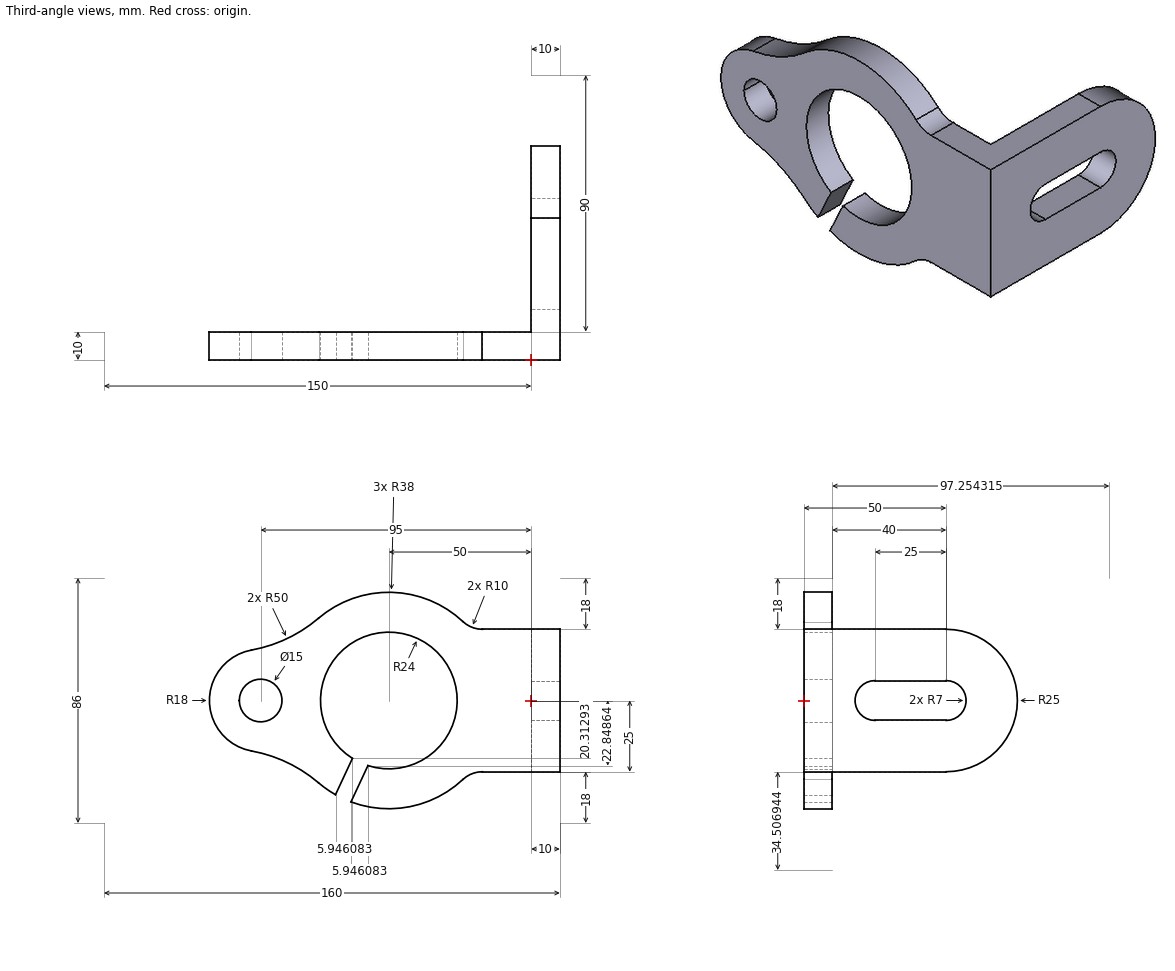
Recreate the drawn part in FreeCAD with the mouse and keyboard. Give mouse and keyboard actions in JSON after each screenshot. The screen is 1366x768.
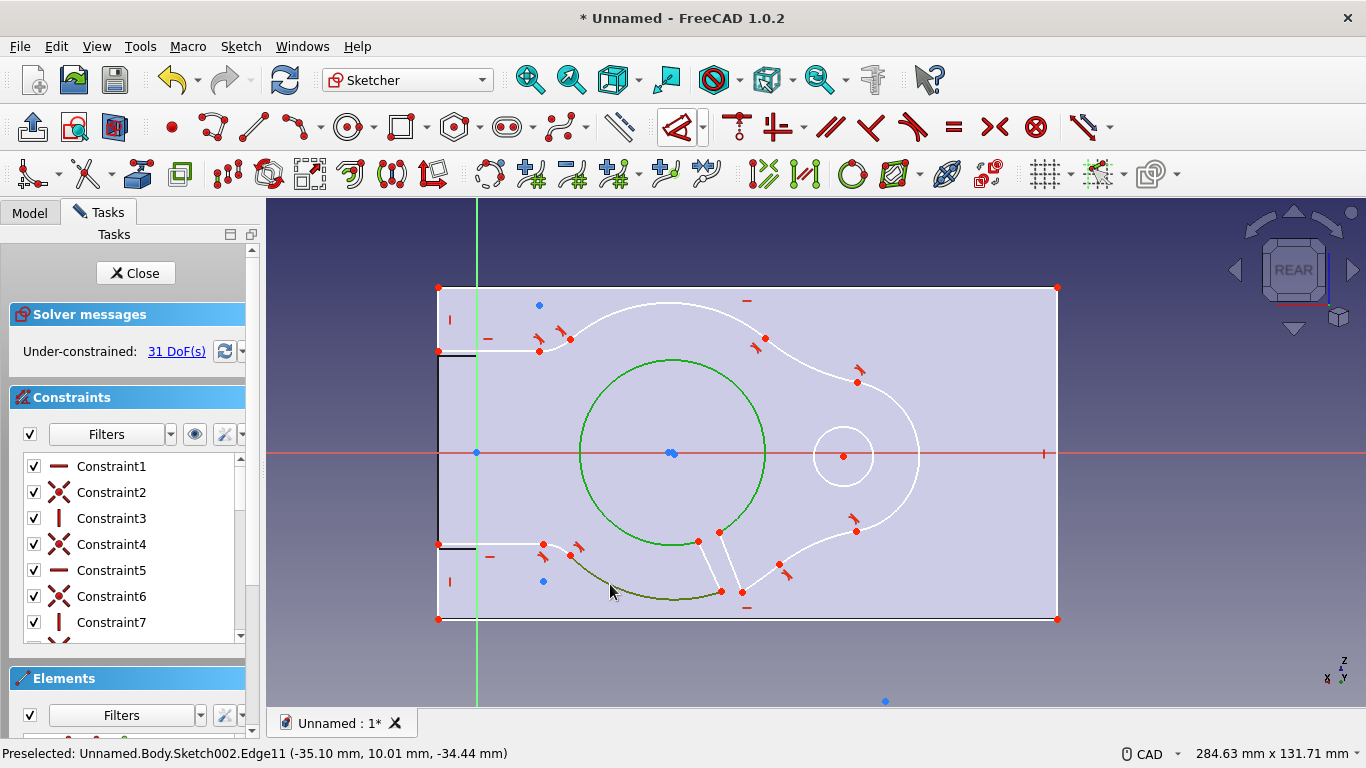
{"action": "left_click", "coordinate": [737, 128]}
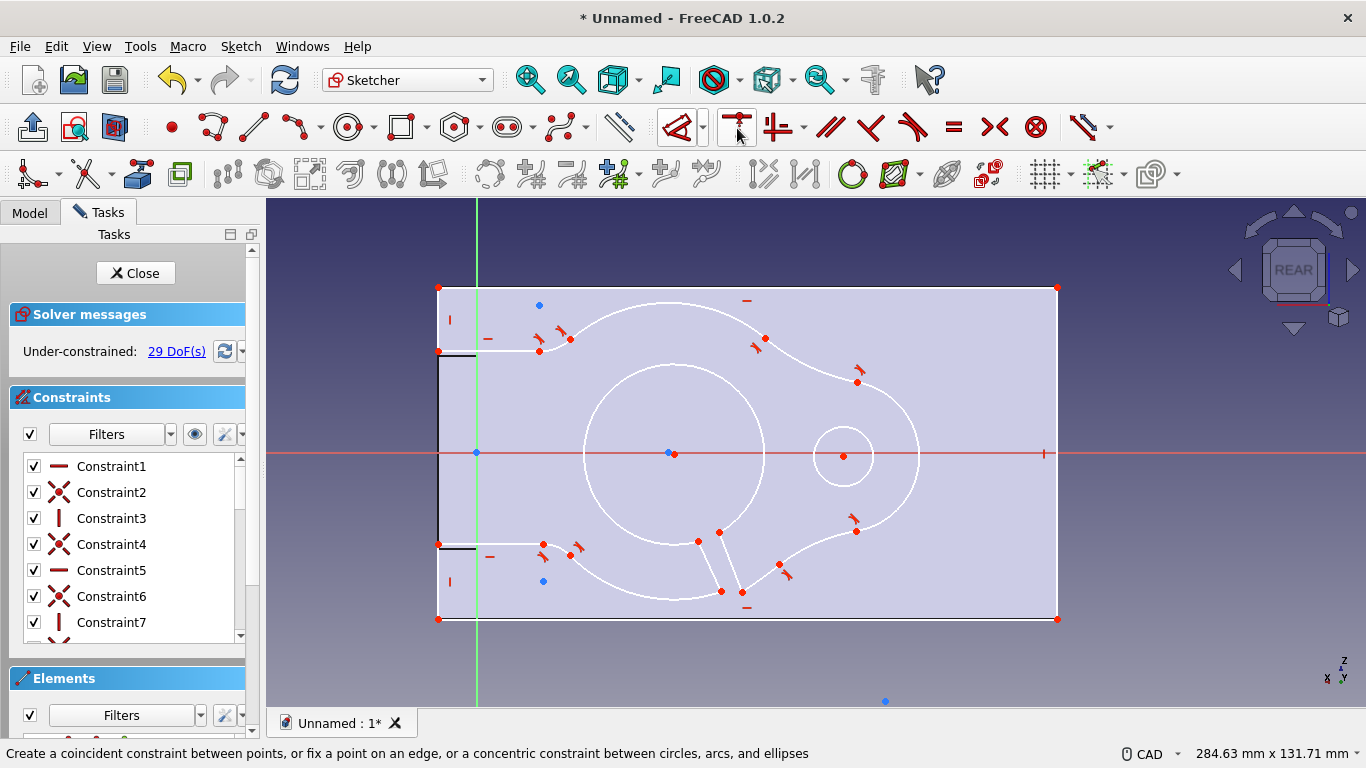
{"action": "left_click", "coordinate": [740, 392]}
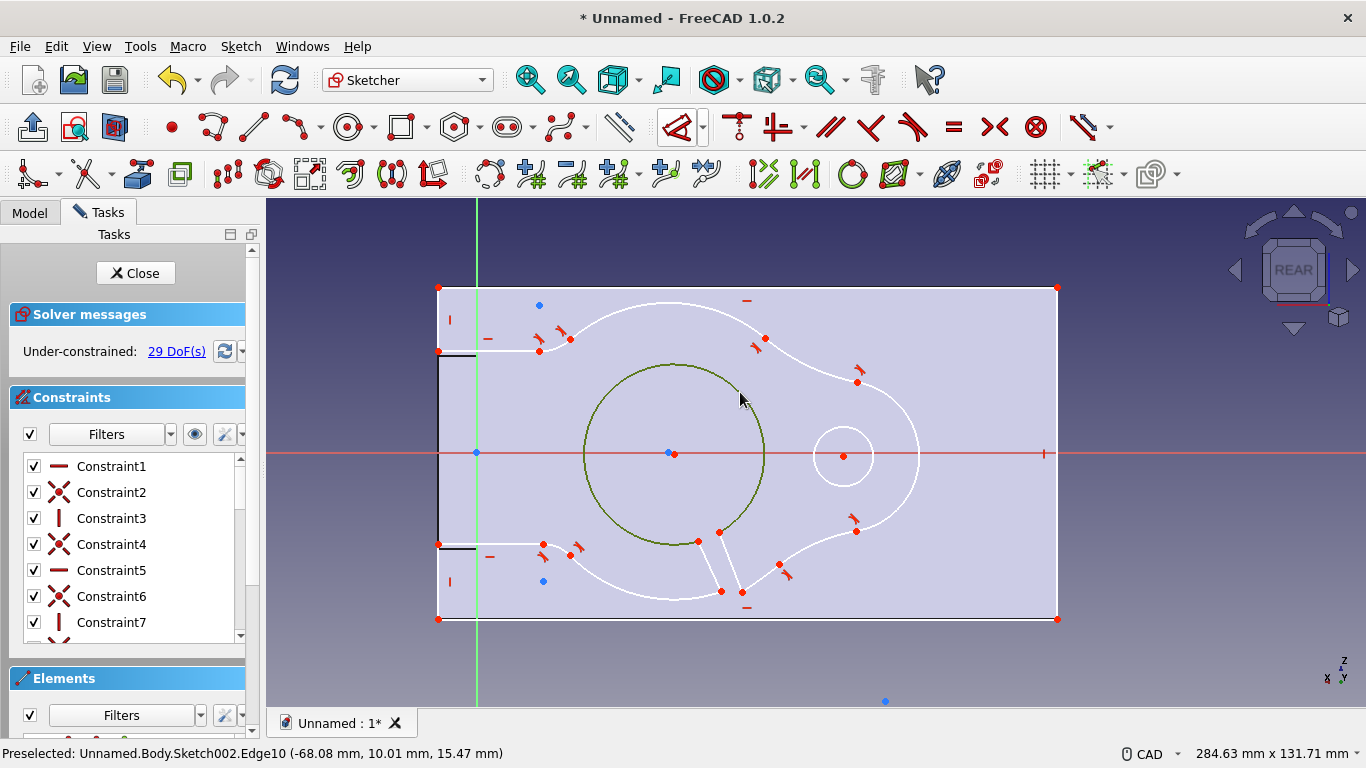
{"action": "left_click", "coordinate": [709, 309]}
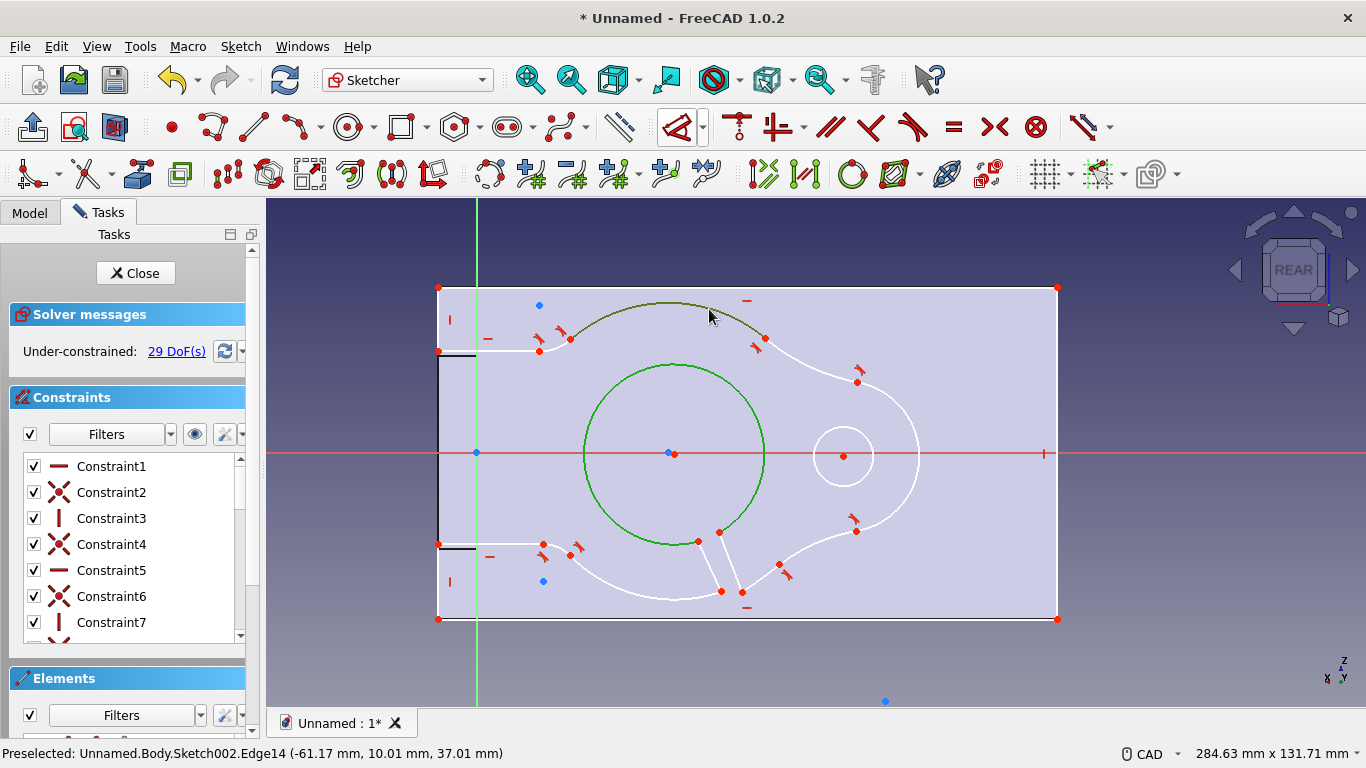
{"action": "key", "text": "c"}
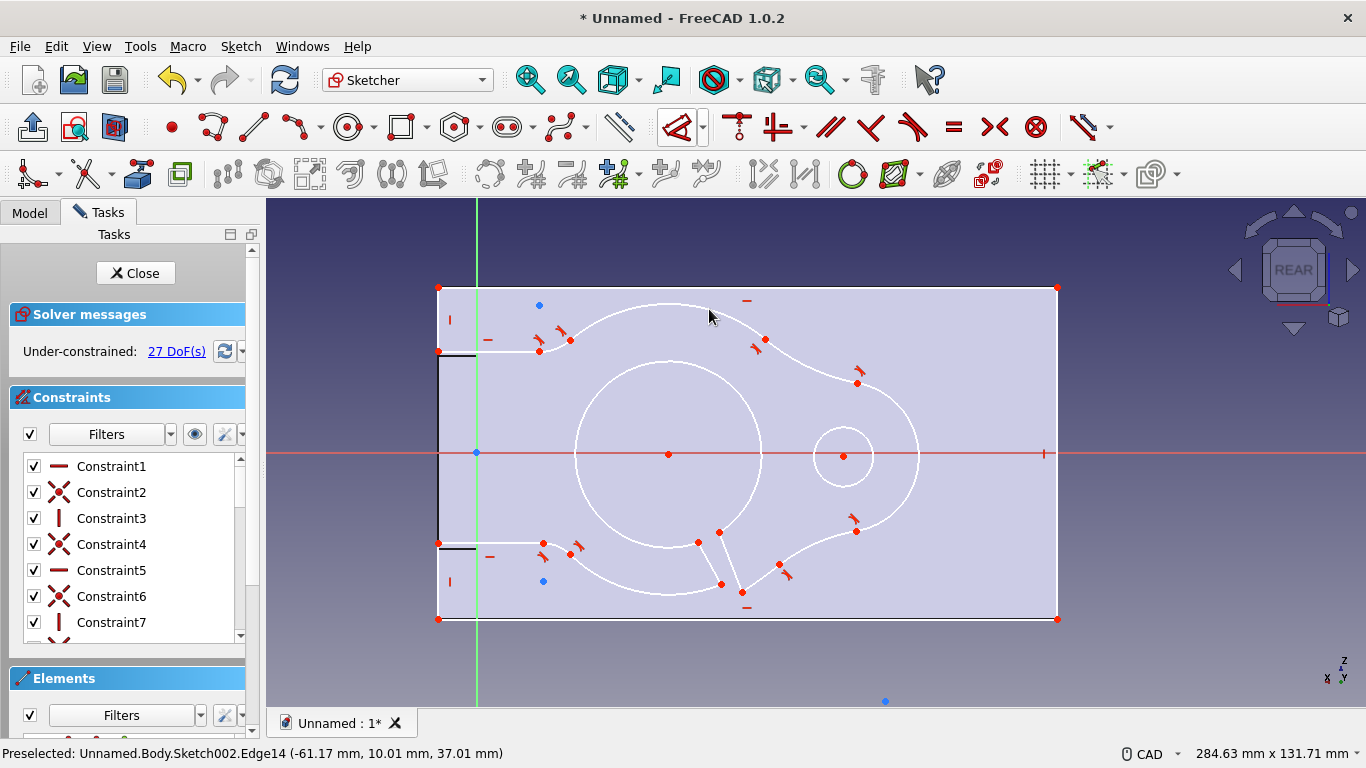
{"action": "left_click", "coordinate": [732, 387]}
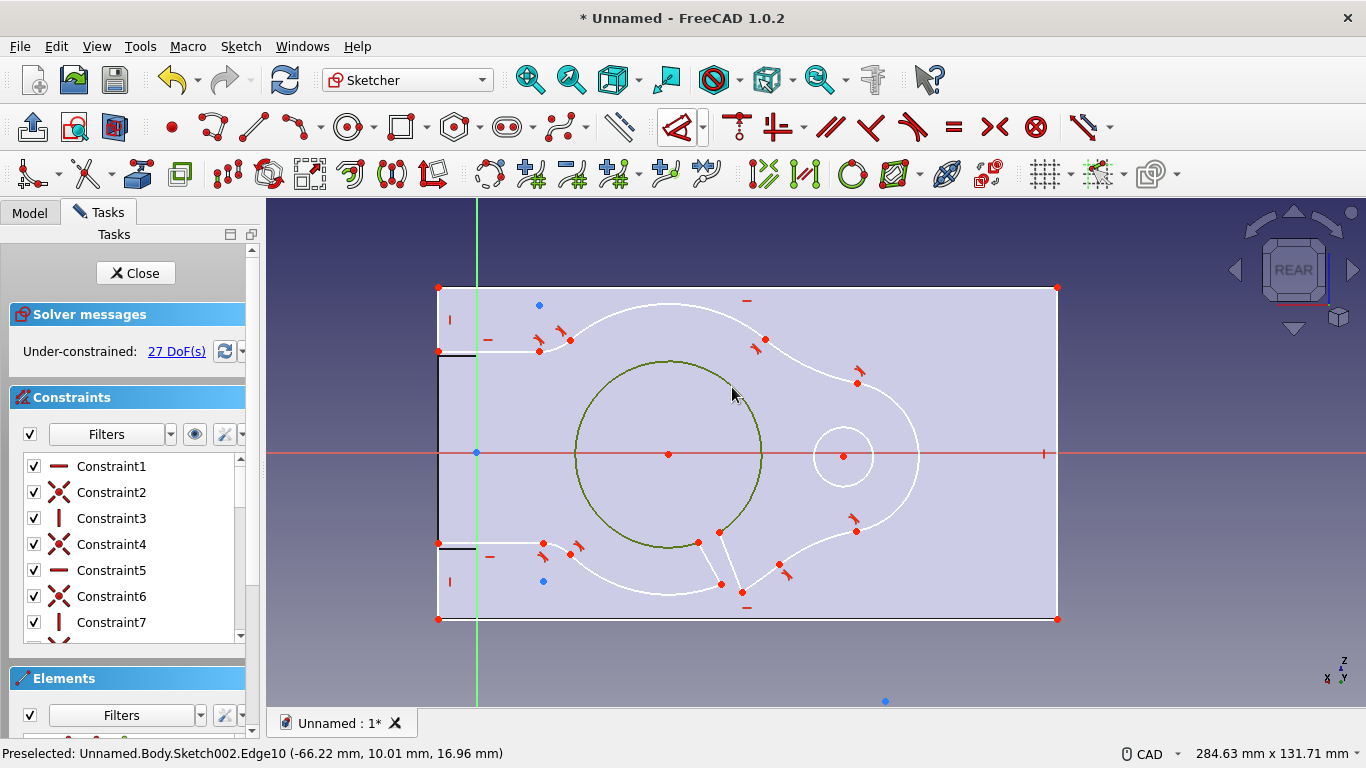
{"action": "left_click", "coordinate": [754, 584]}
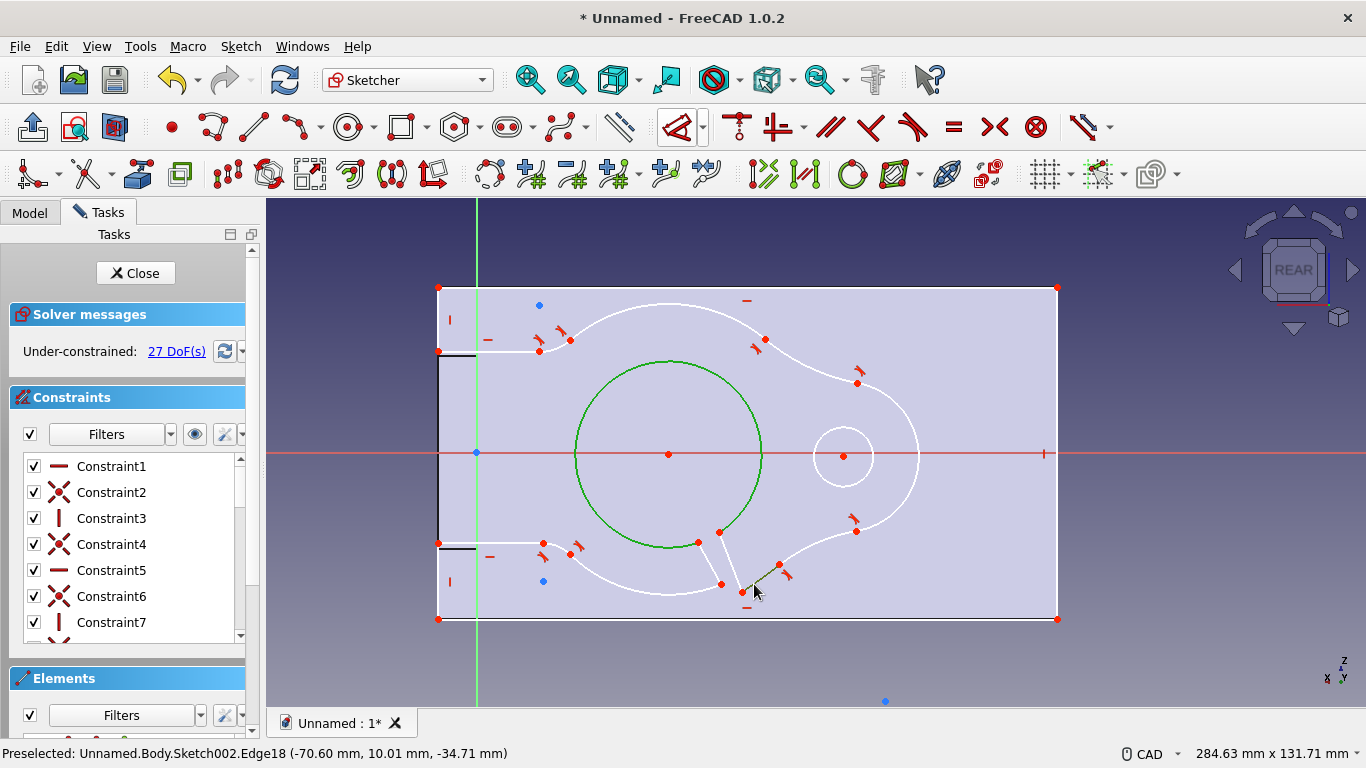
{"action": "left_click", "coordinate": [737, 128]}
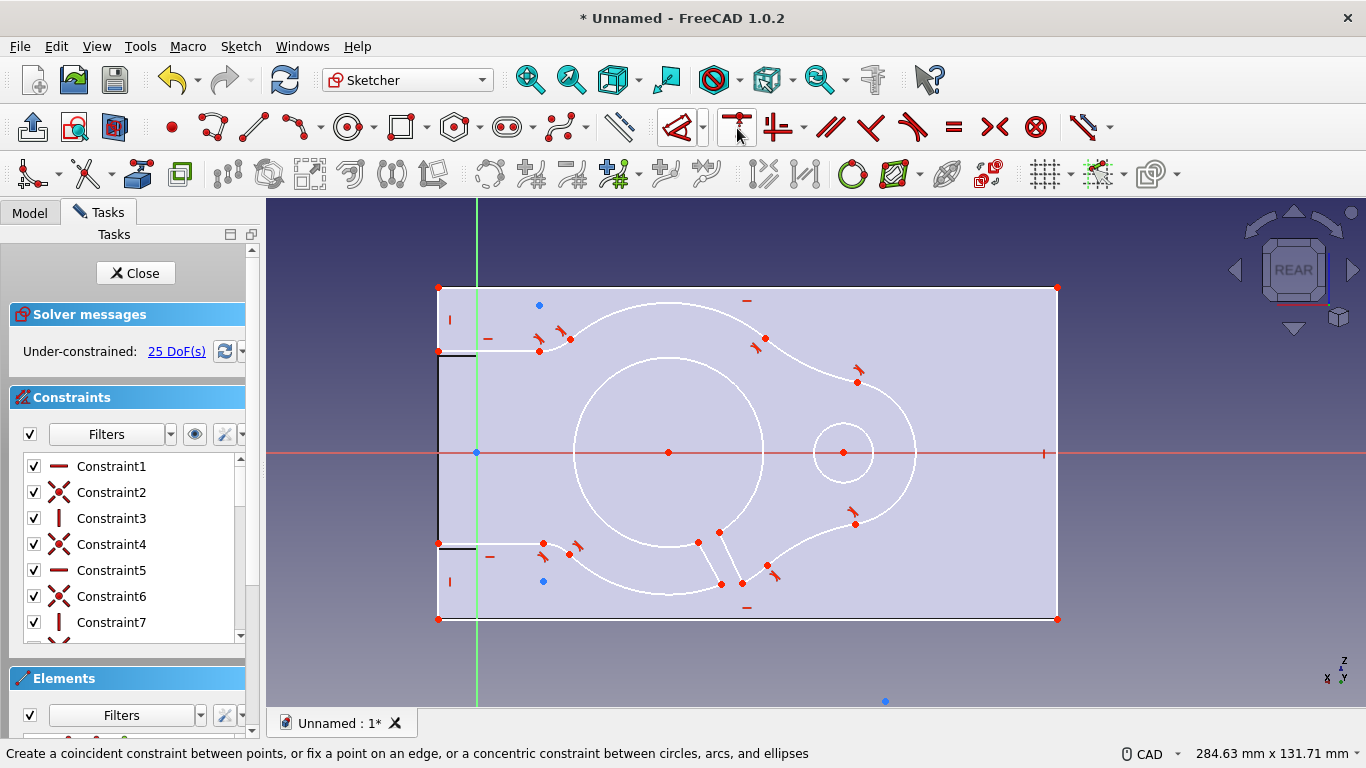
{"action": "left_click", "coordinate": [557, 546]}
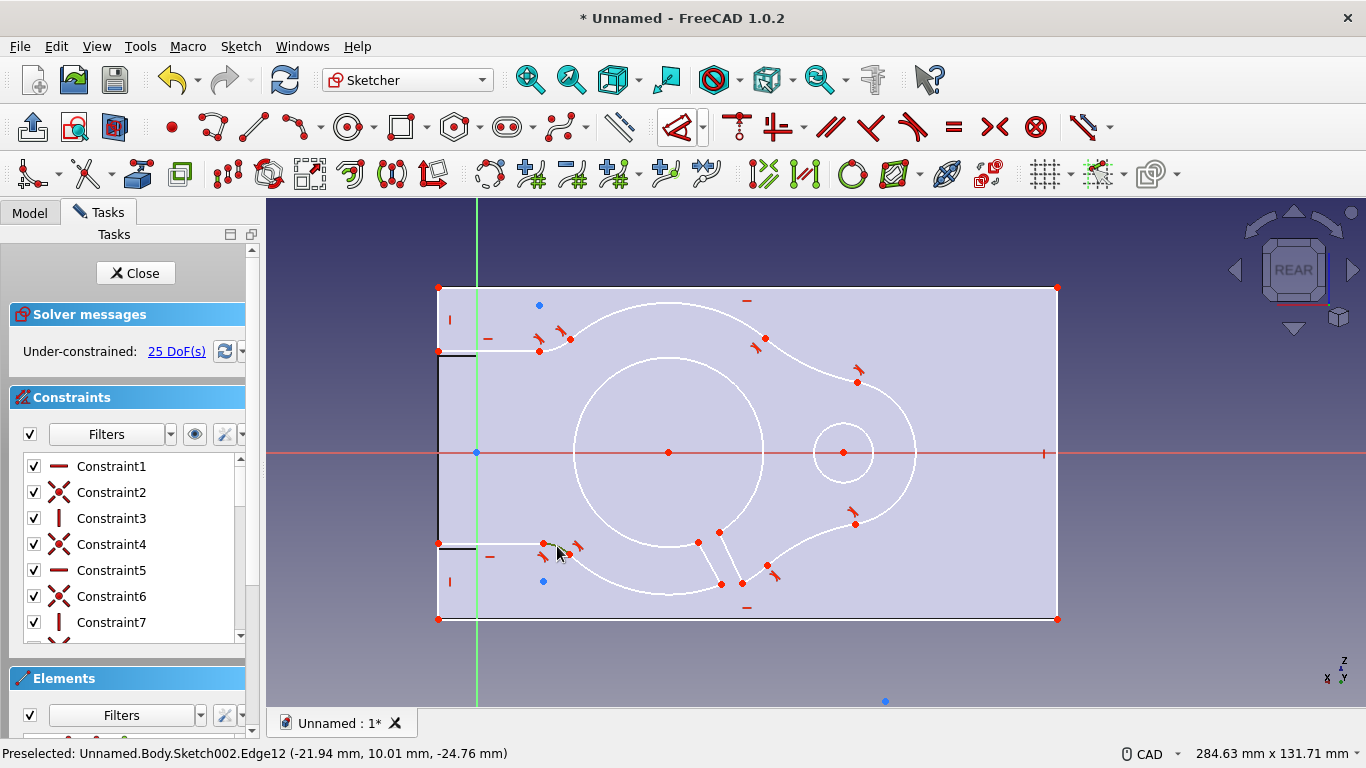
{"action": "scroll", "coordinate": [550, 350], "scroll_direction": "up", "scroll_amount": 2}